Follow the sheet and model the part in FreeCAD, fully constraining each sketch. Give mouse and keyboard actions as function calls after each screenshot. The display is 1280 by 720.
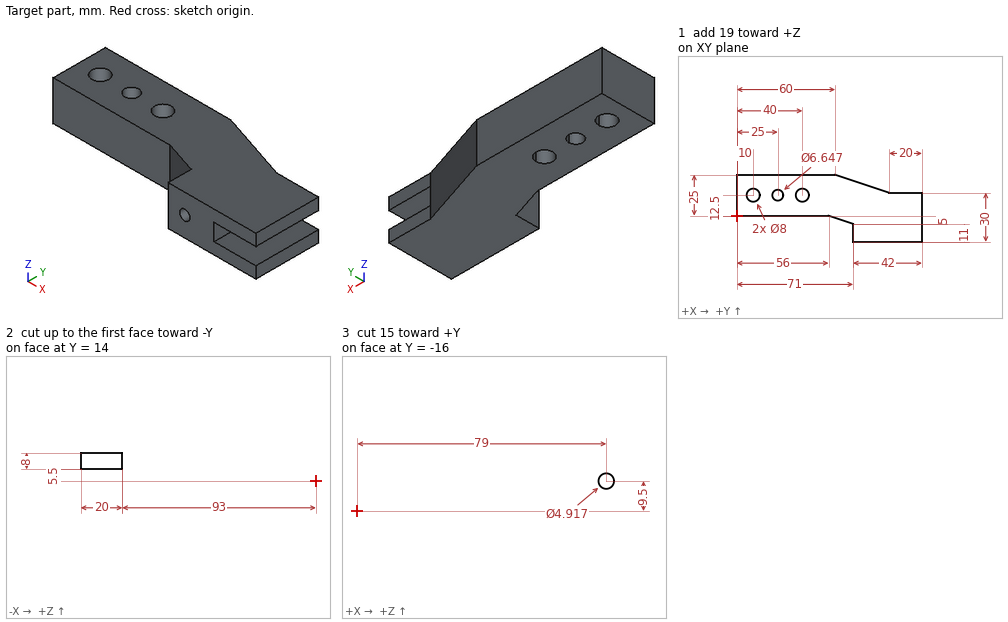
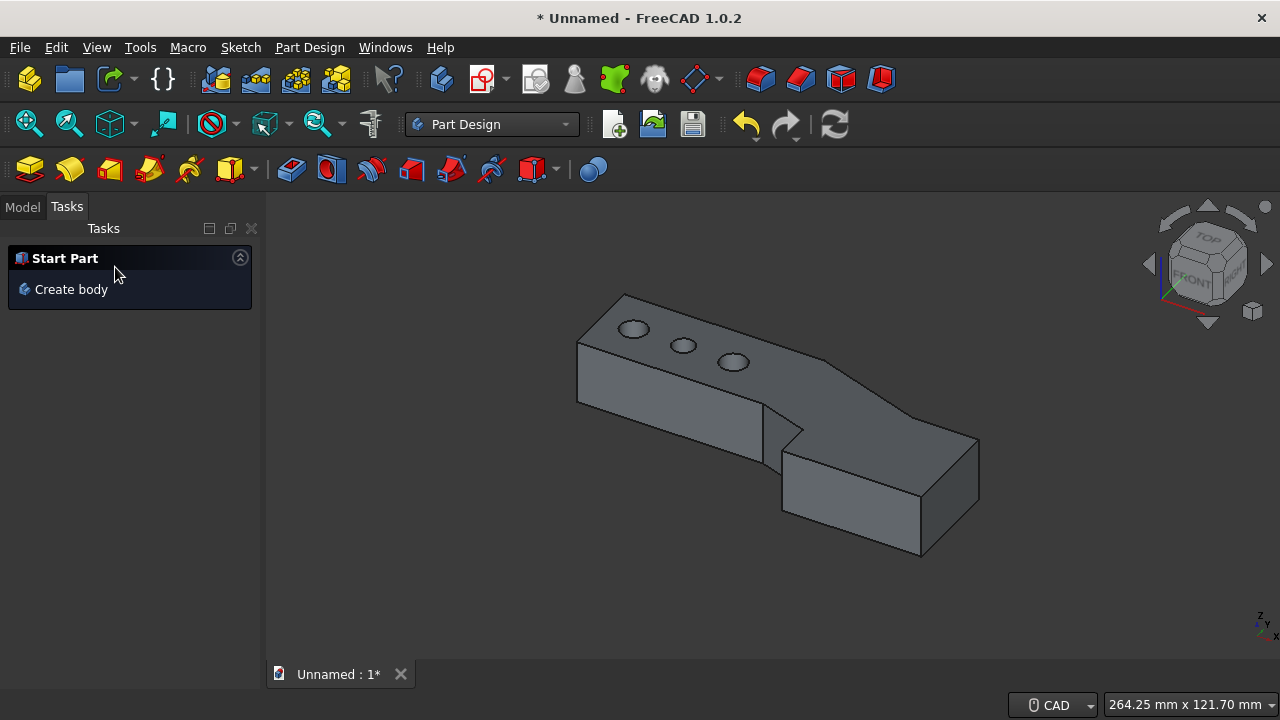
key(4)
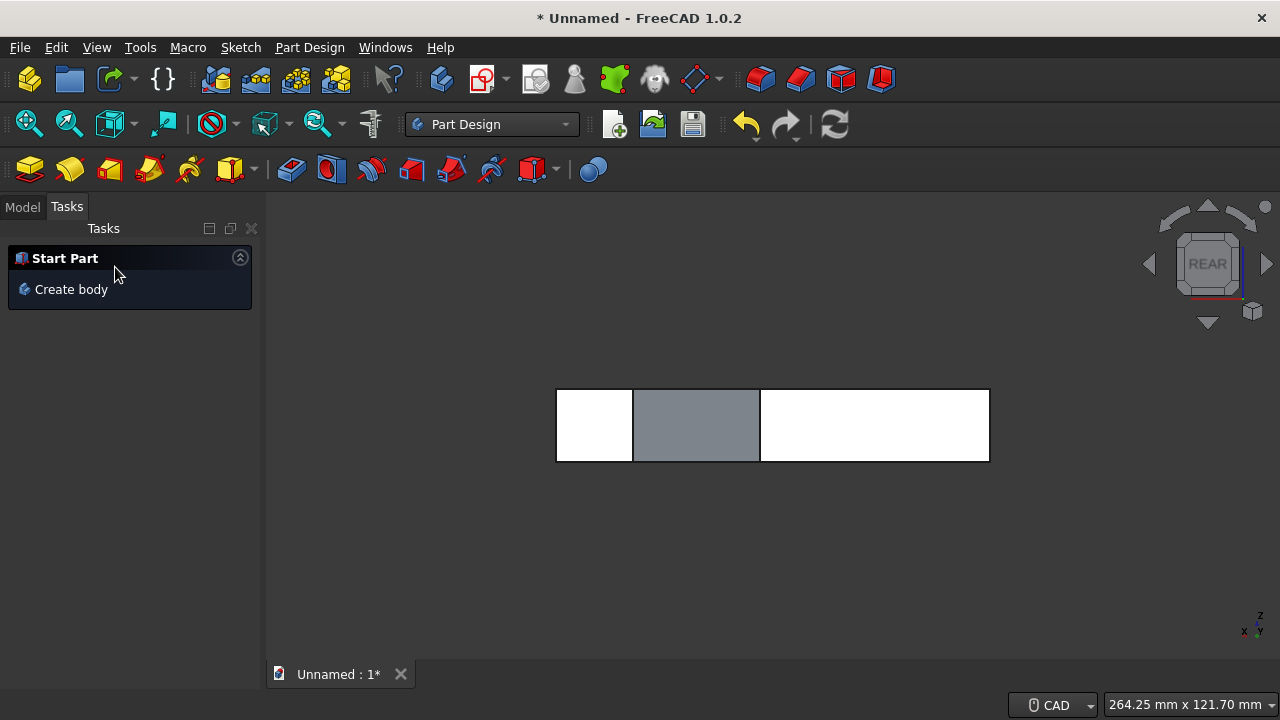
click(30, 124)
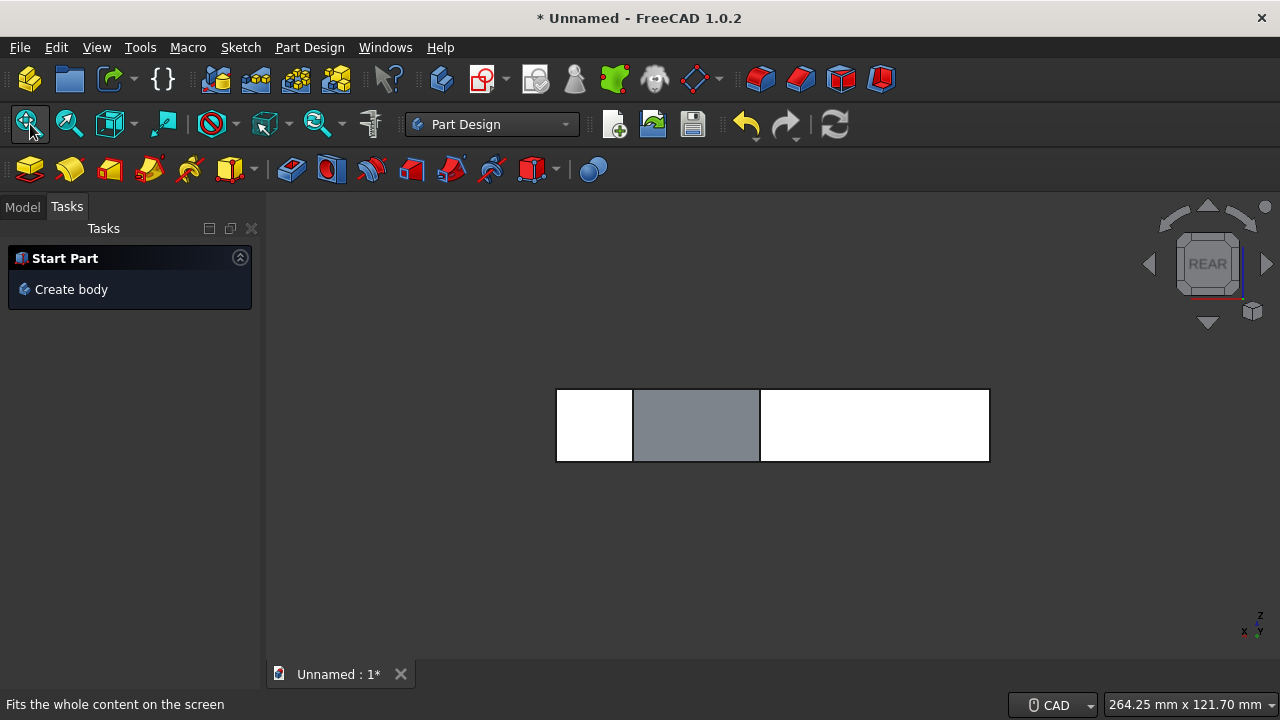
click(595, 425)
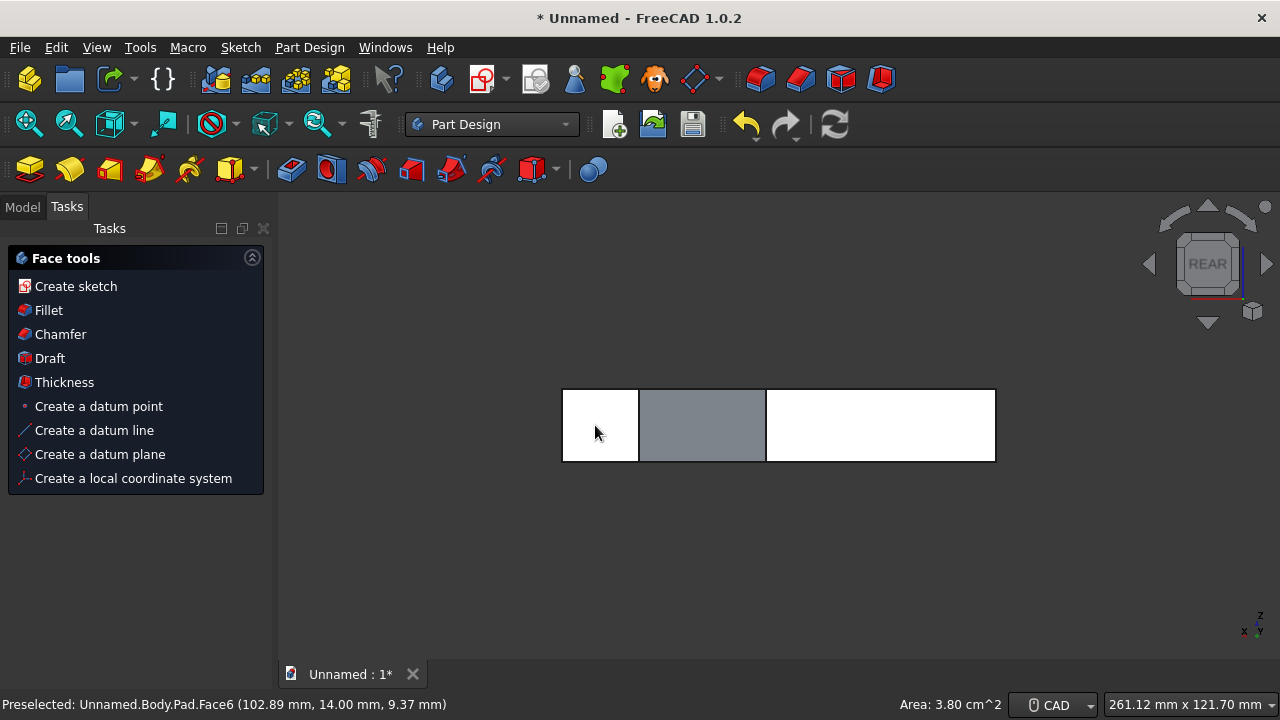
click(482, 80)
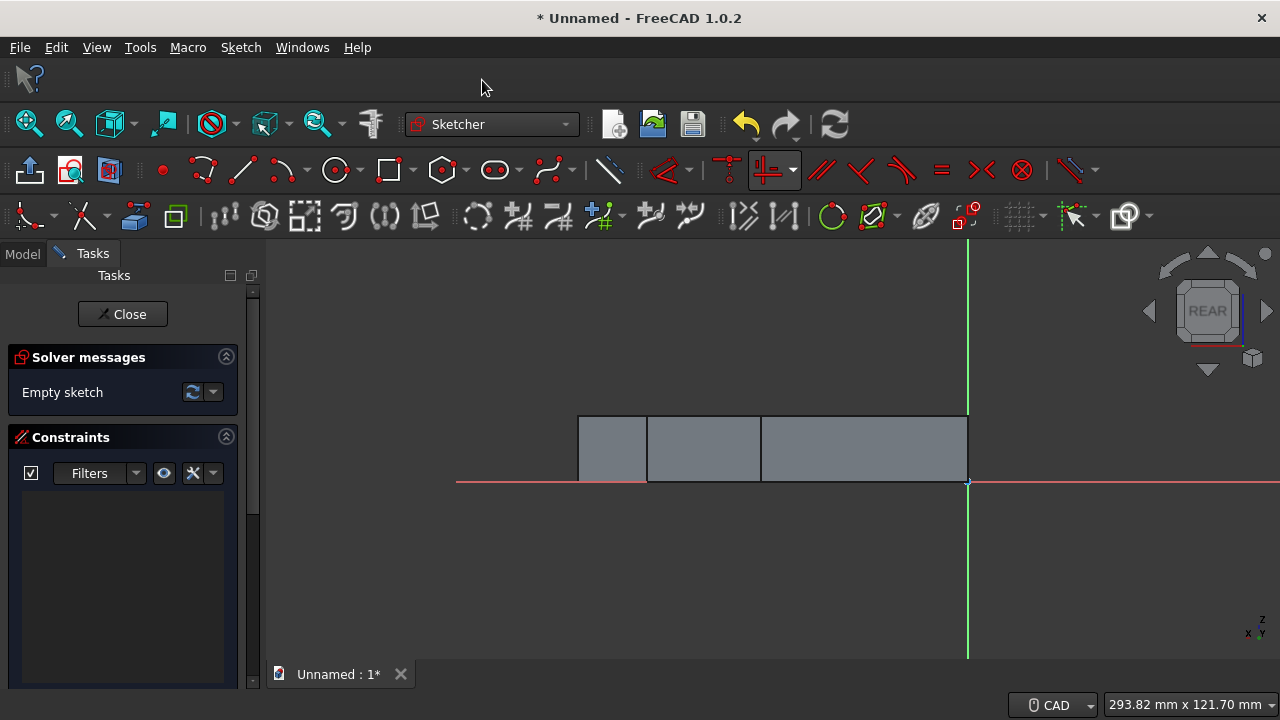
scroll(601, 449, up, 11)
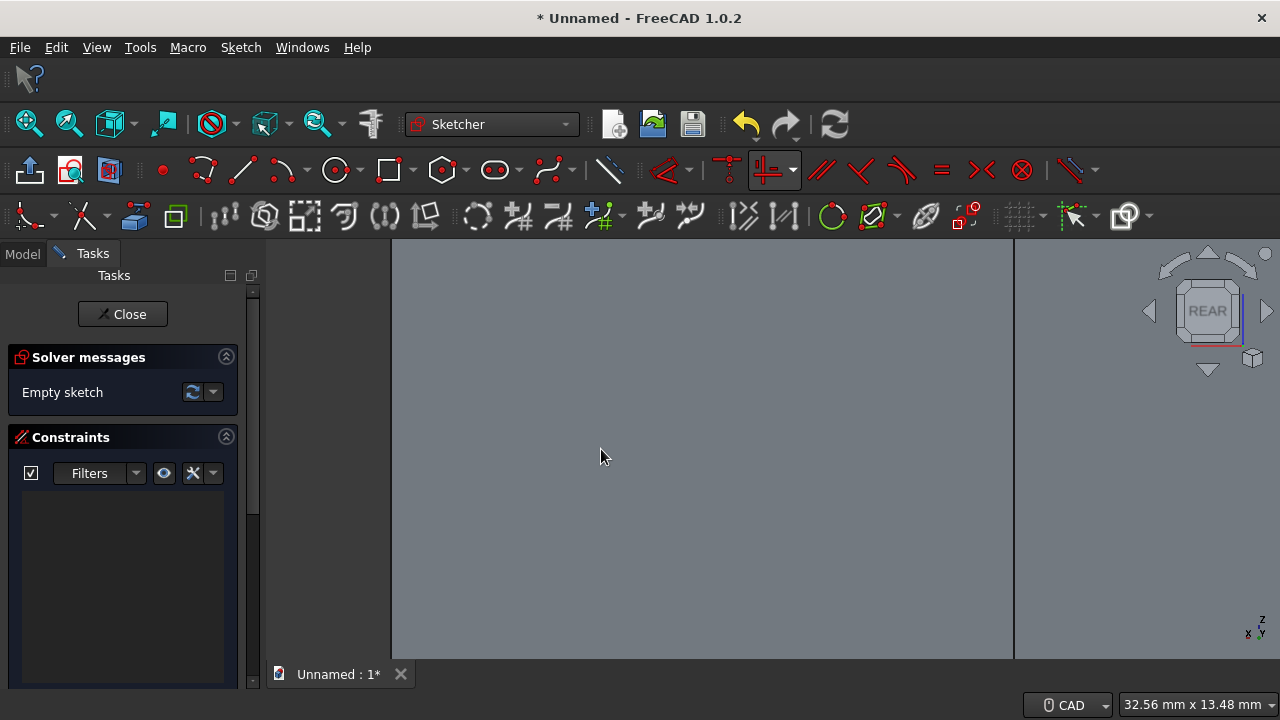
key(g)
key(r)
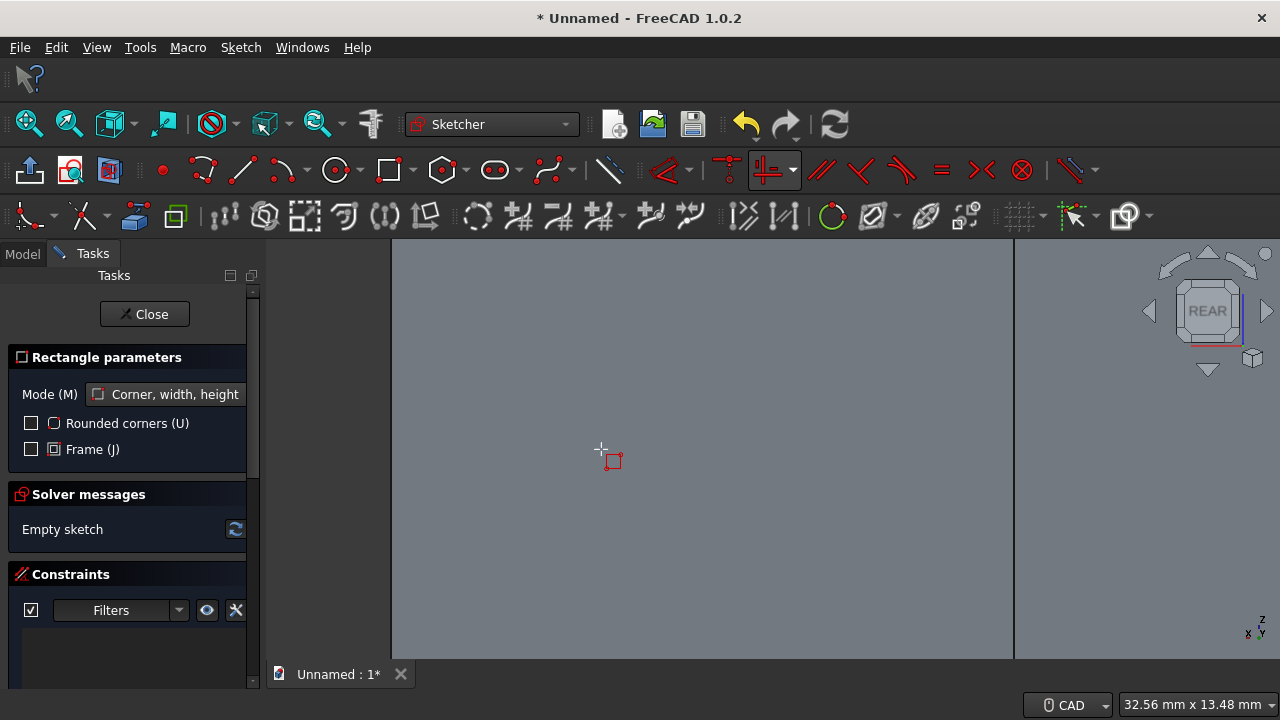
click(391, 320)
click(1014, 570)
key(Escape)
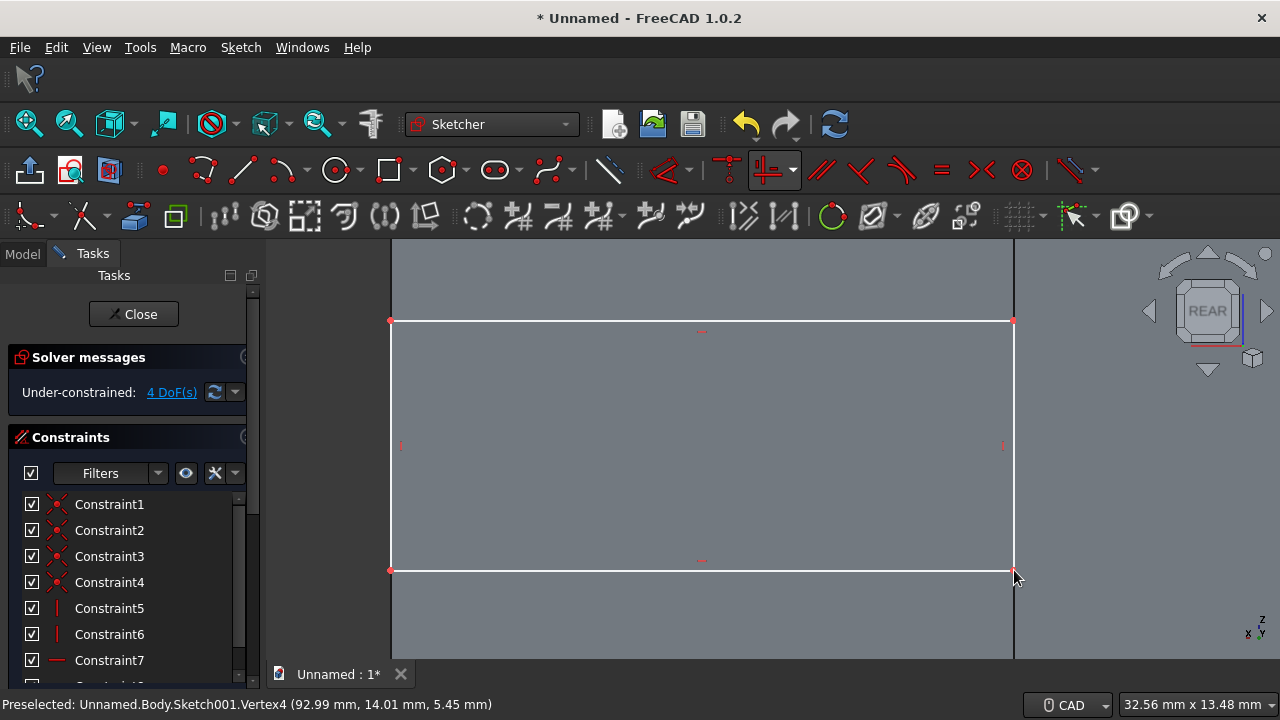
click(664, 170)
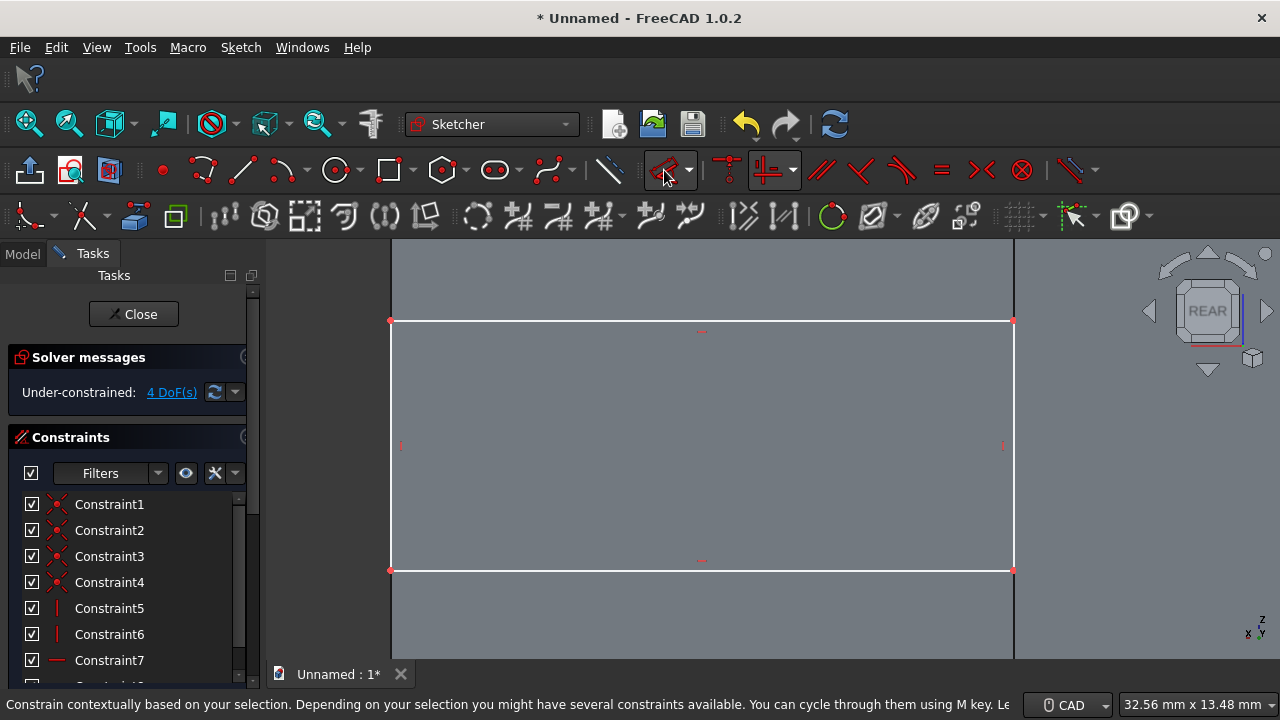
click(391, 396)
click(357, 446)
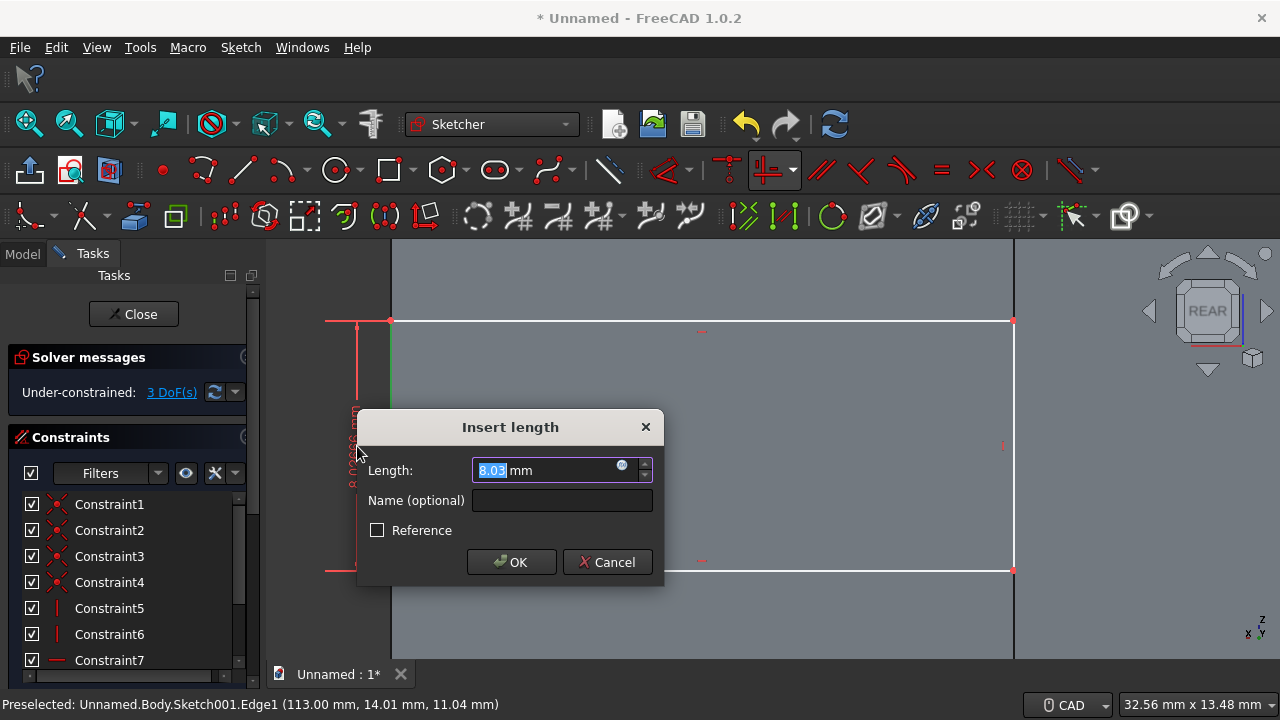
text(8)
key(Return)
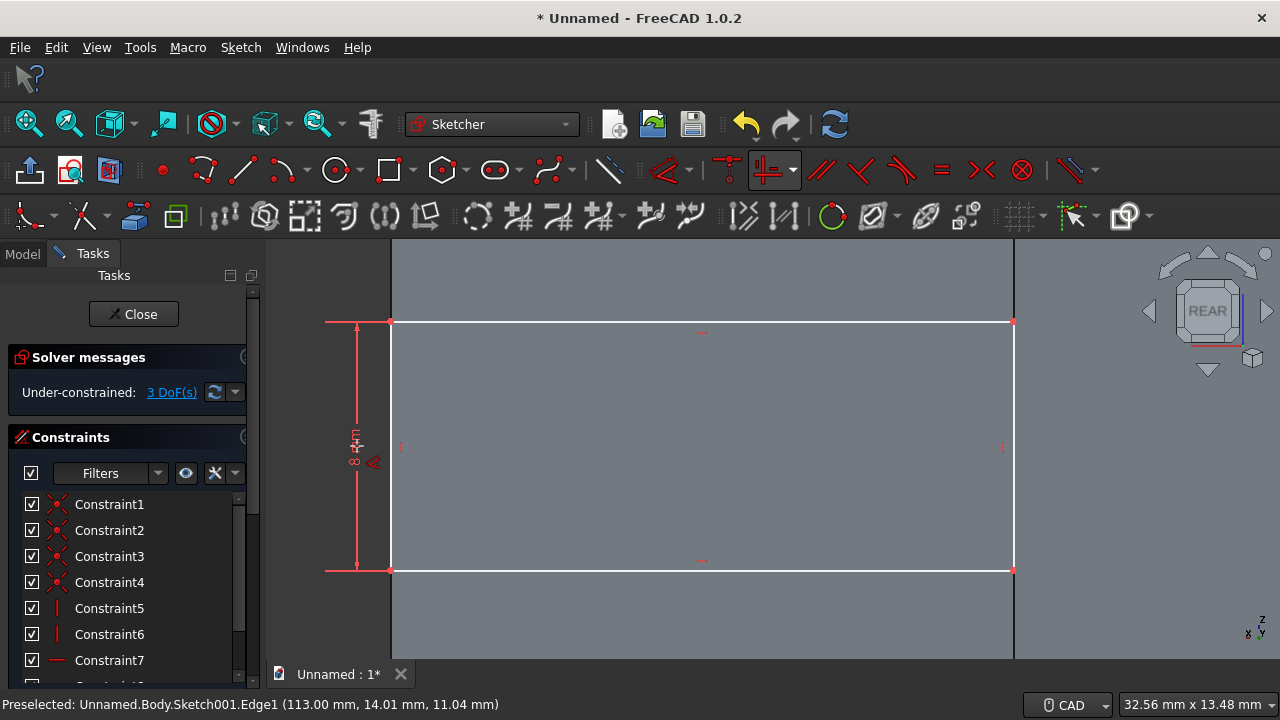
click(578, 571)
click(702, 605)